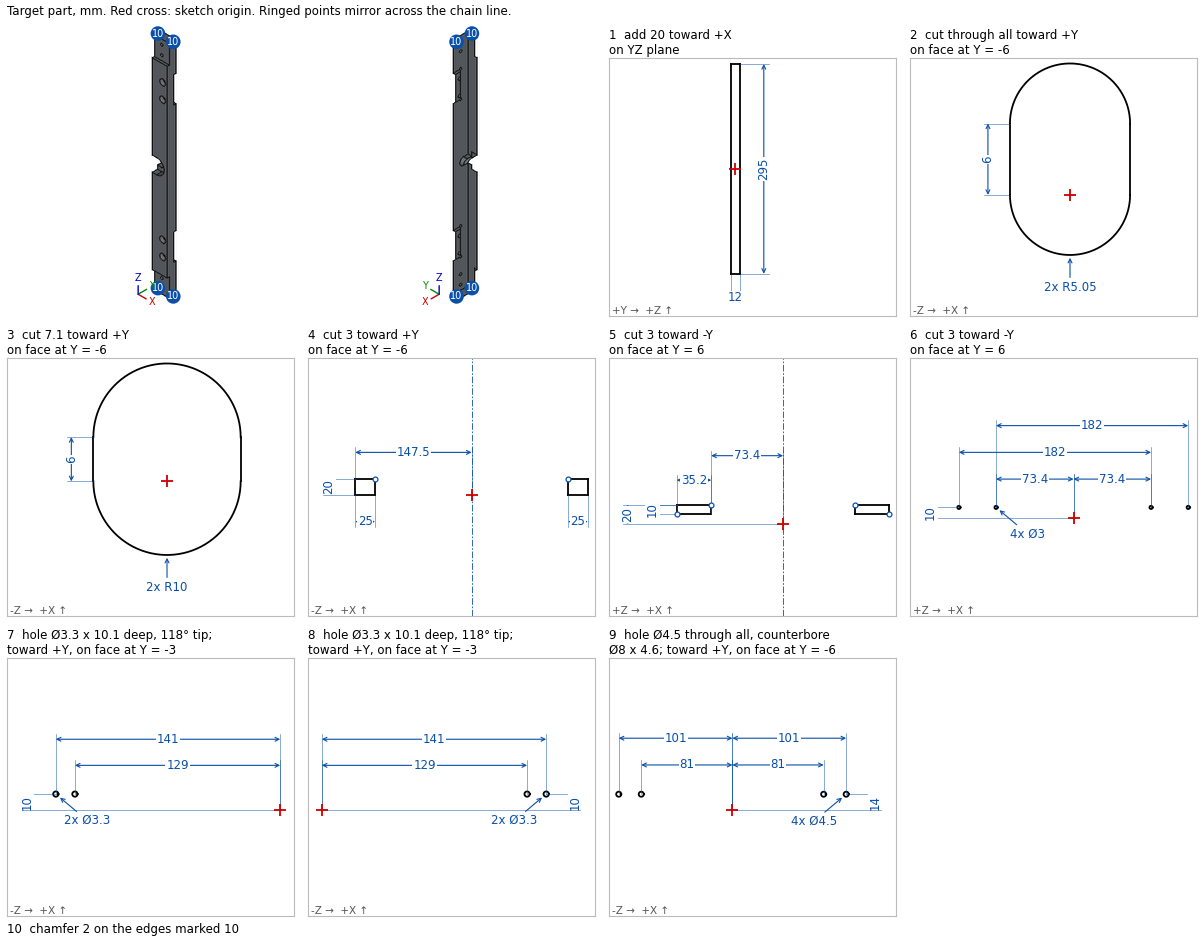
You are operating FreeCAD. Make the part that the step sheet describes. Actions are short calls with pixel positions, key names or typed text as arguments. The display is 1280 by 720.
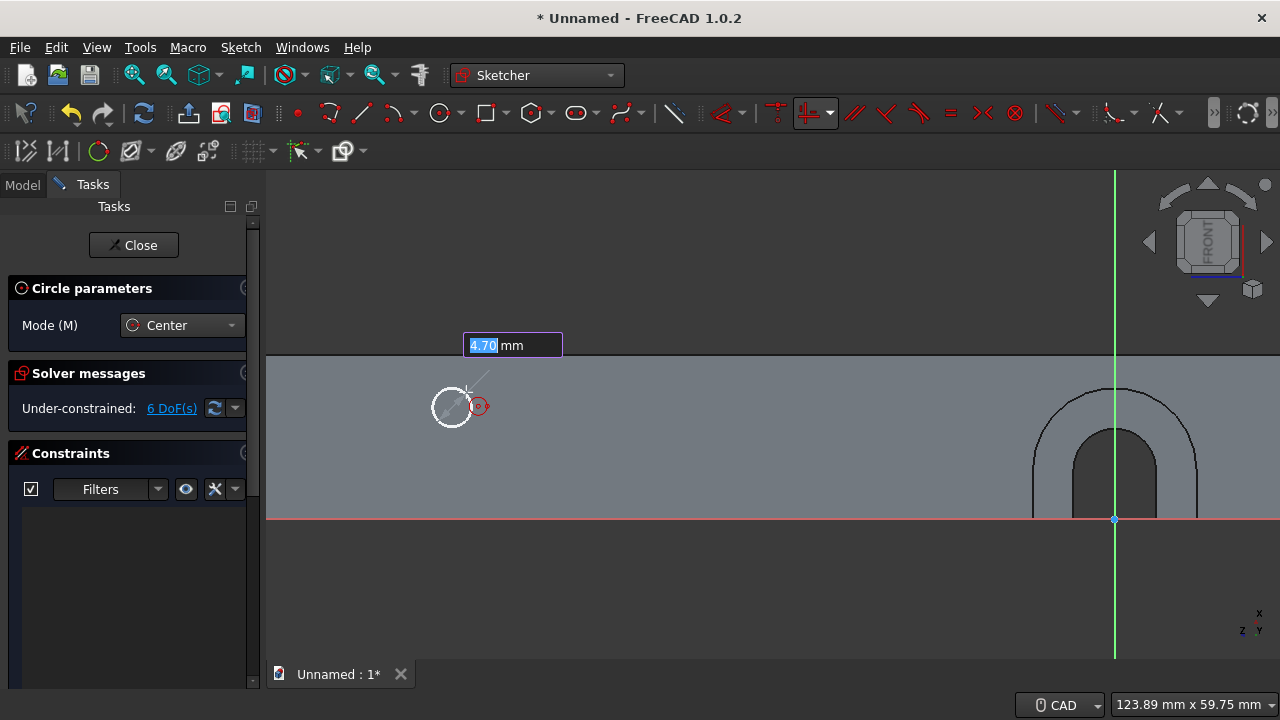
click(465, 391)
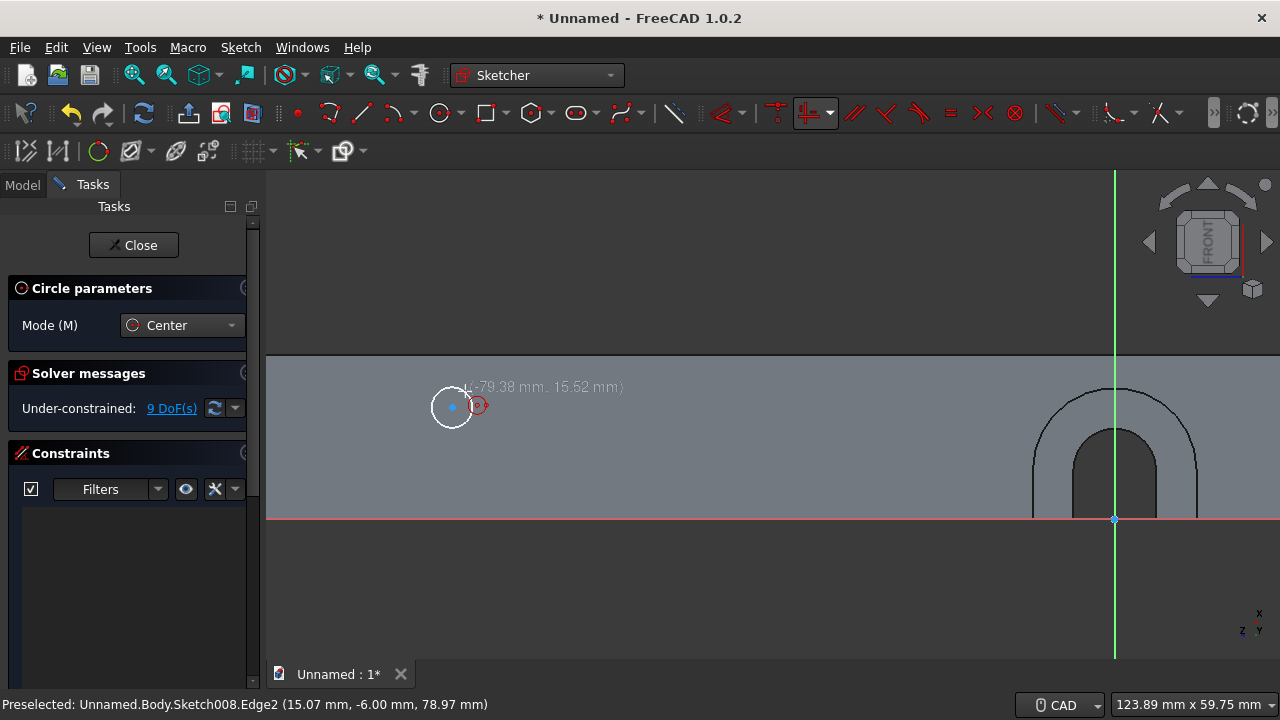
scroll(466, 392, down, 5)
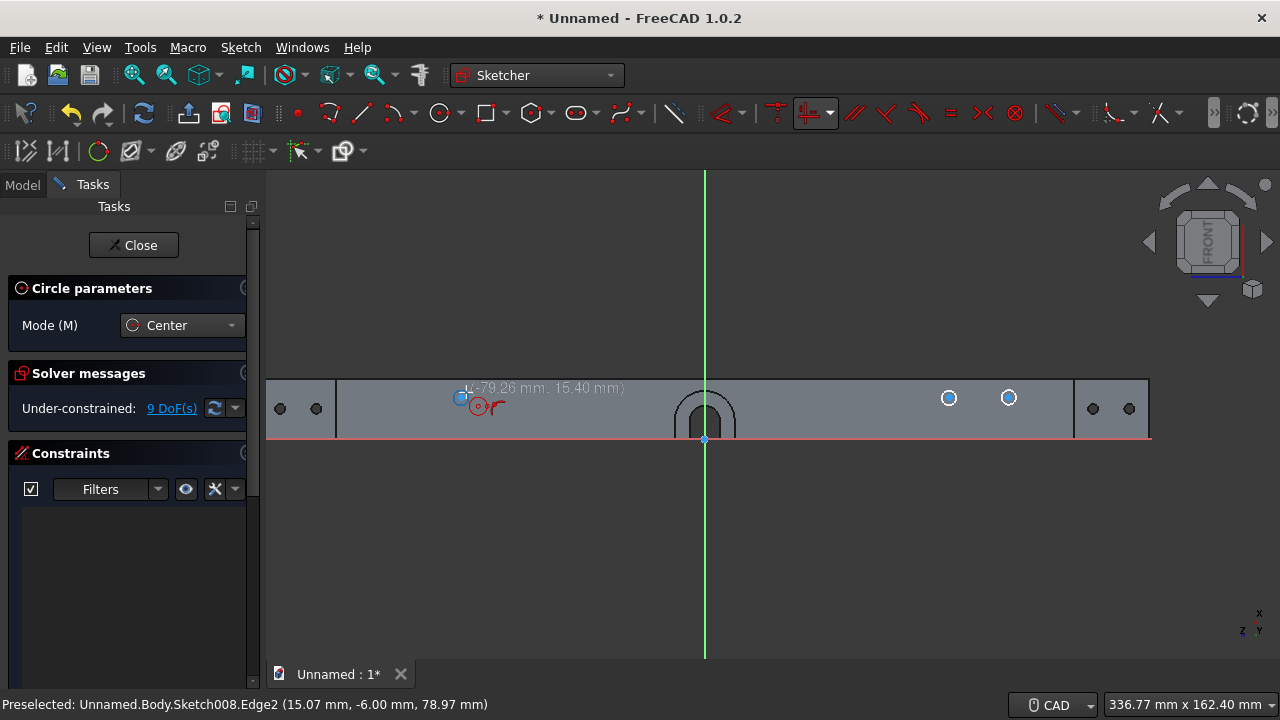
scroll(401, 397, up, 7)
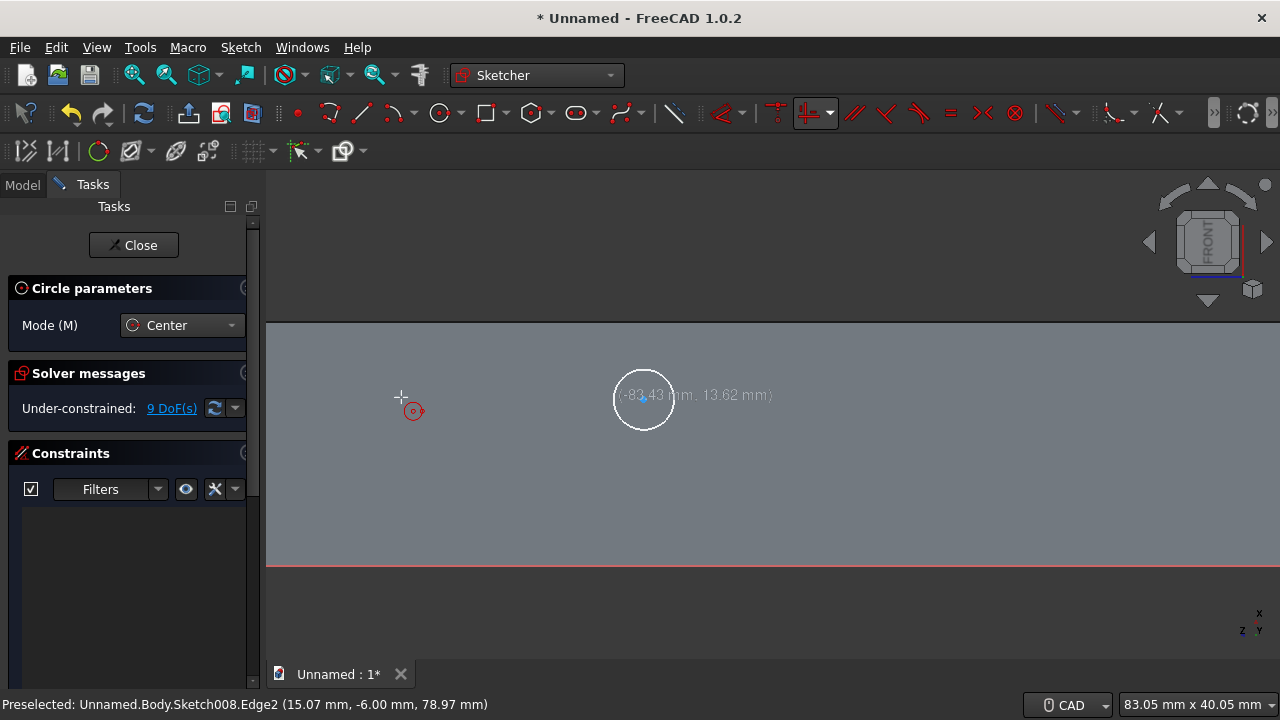
scroll(401, 397, down, 7)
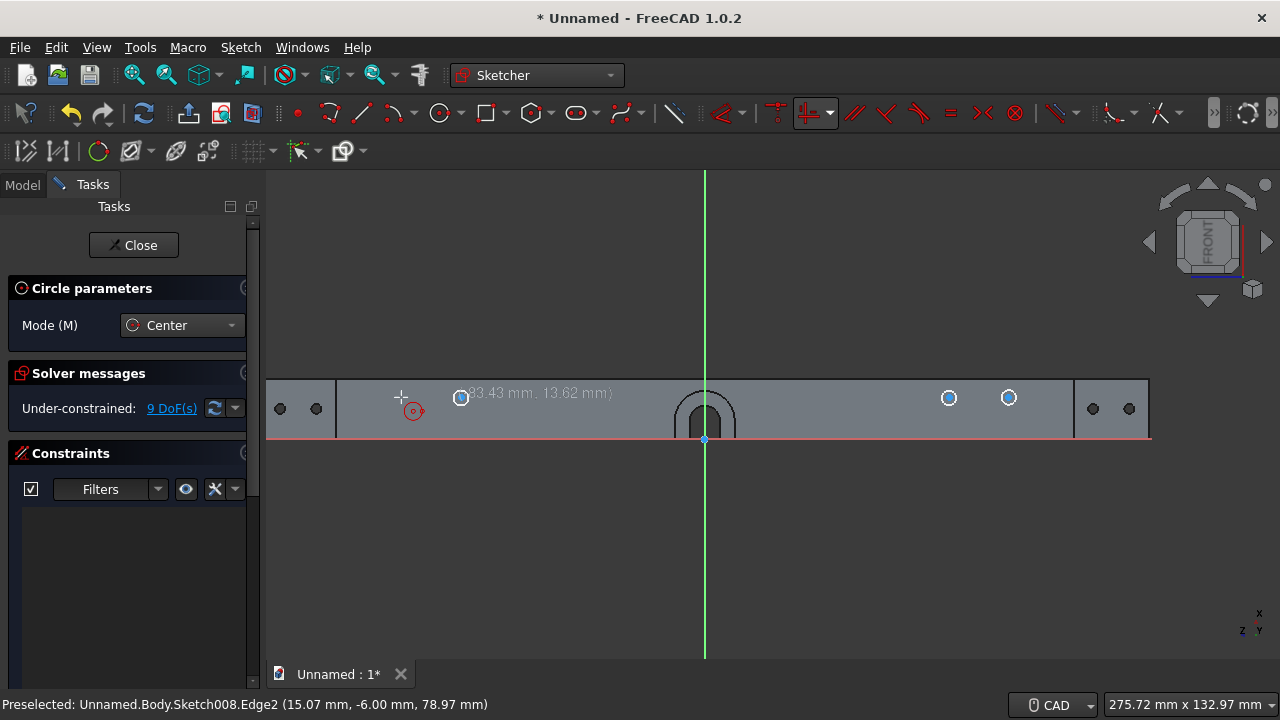
click(401, 397)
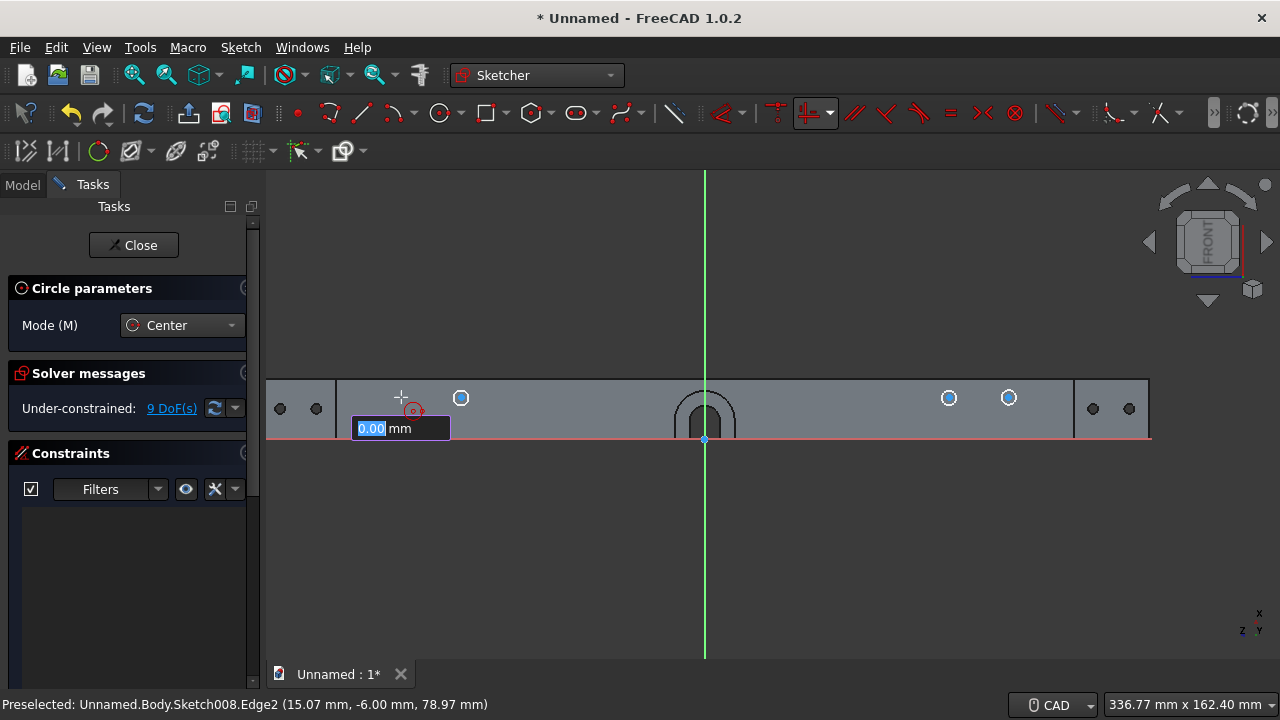
scroll(405, 392, up, 5)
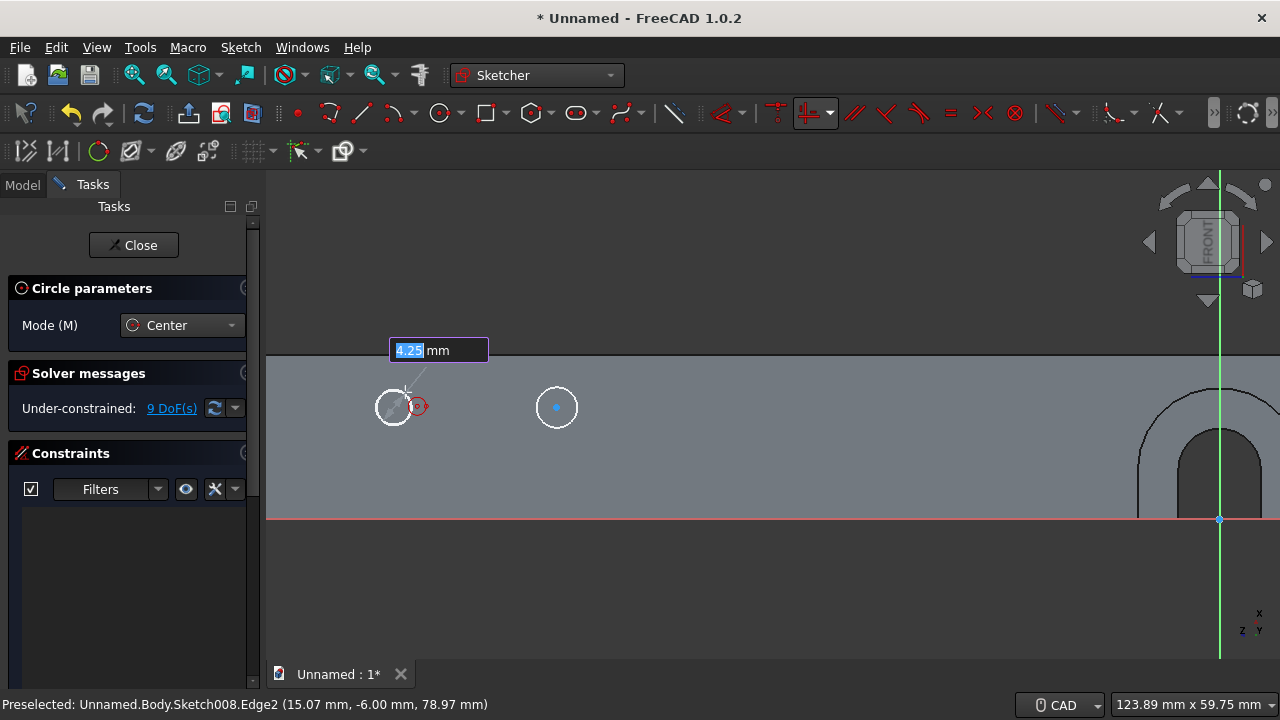
click(406, 391)
key(Escape)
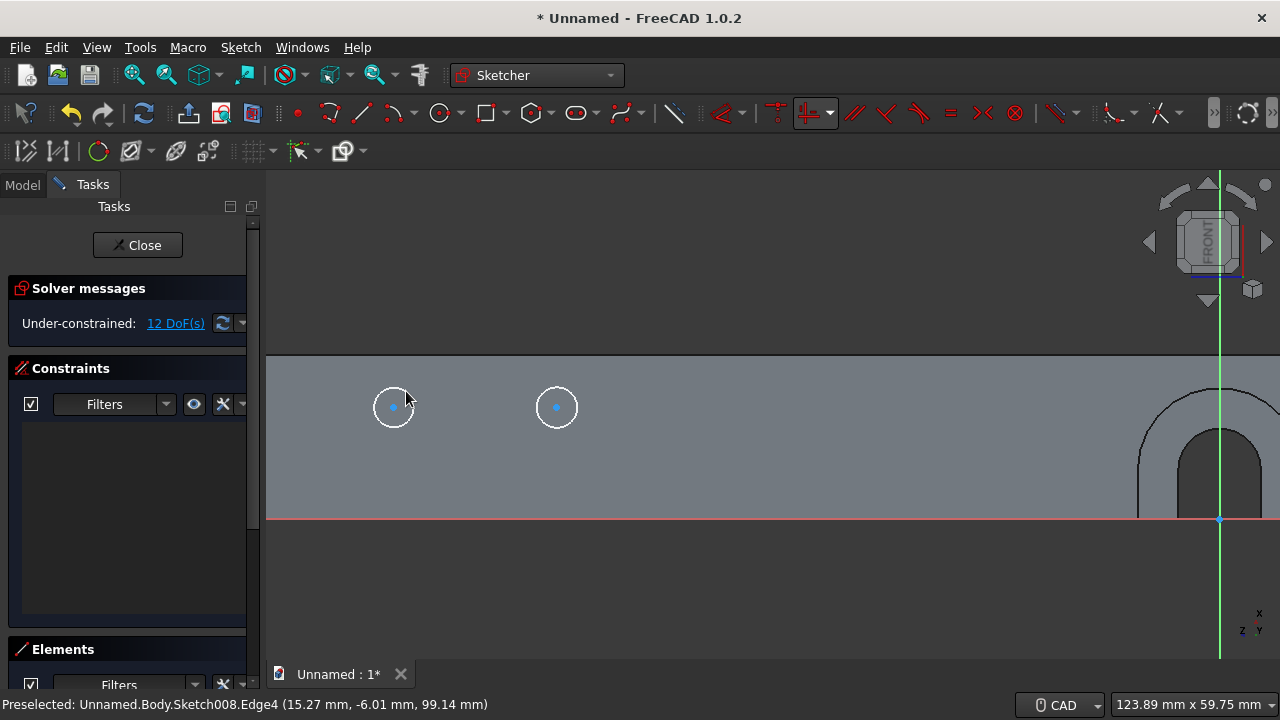
scroll(405, 392, down, 5)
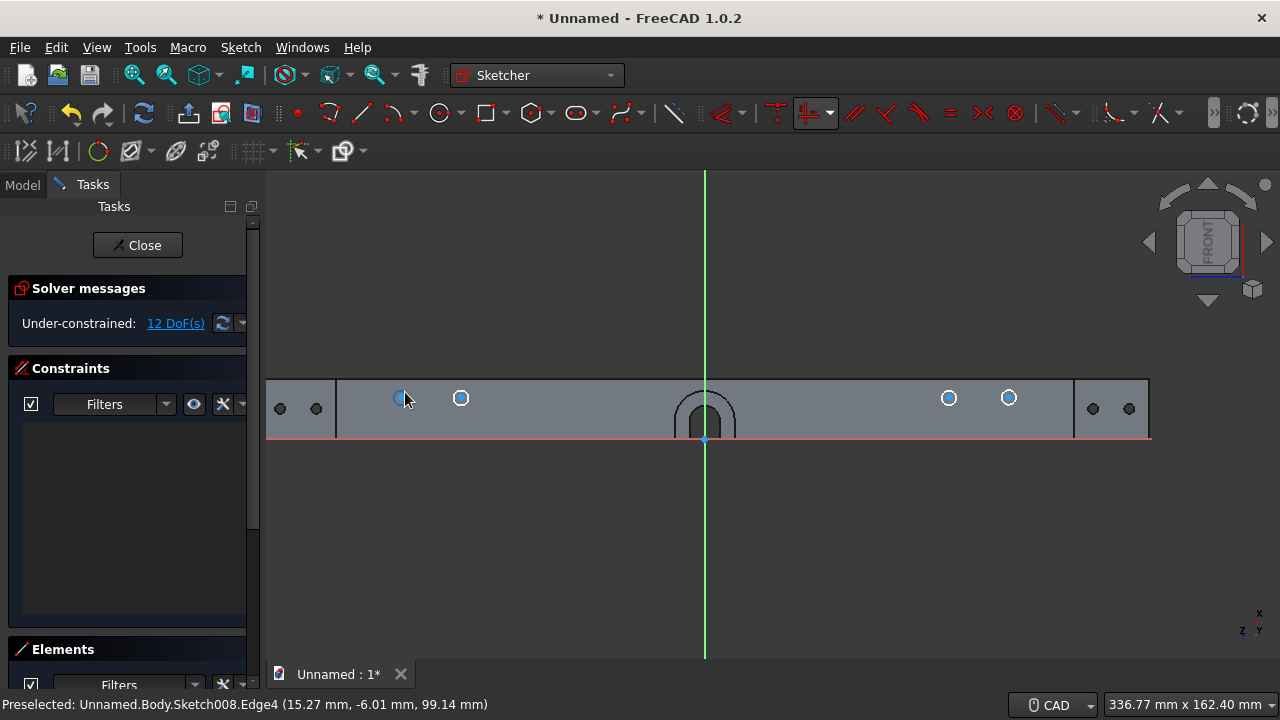
scroll(1014, 392, up, 4)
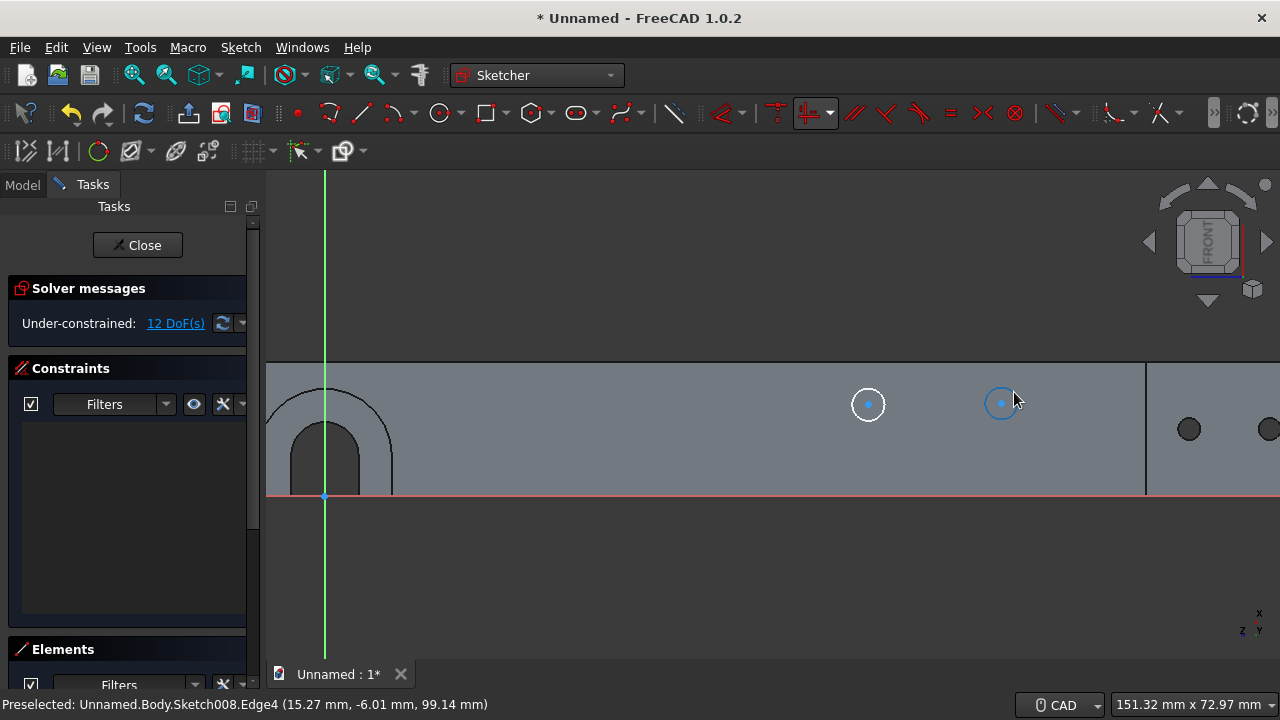
click(1013, 392)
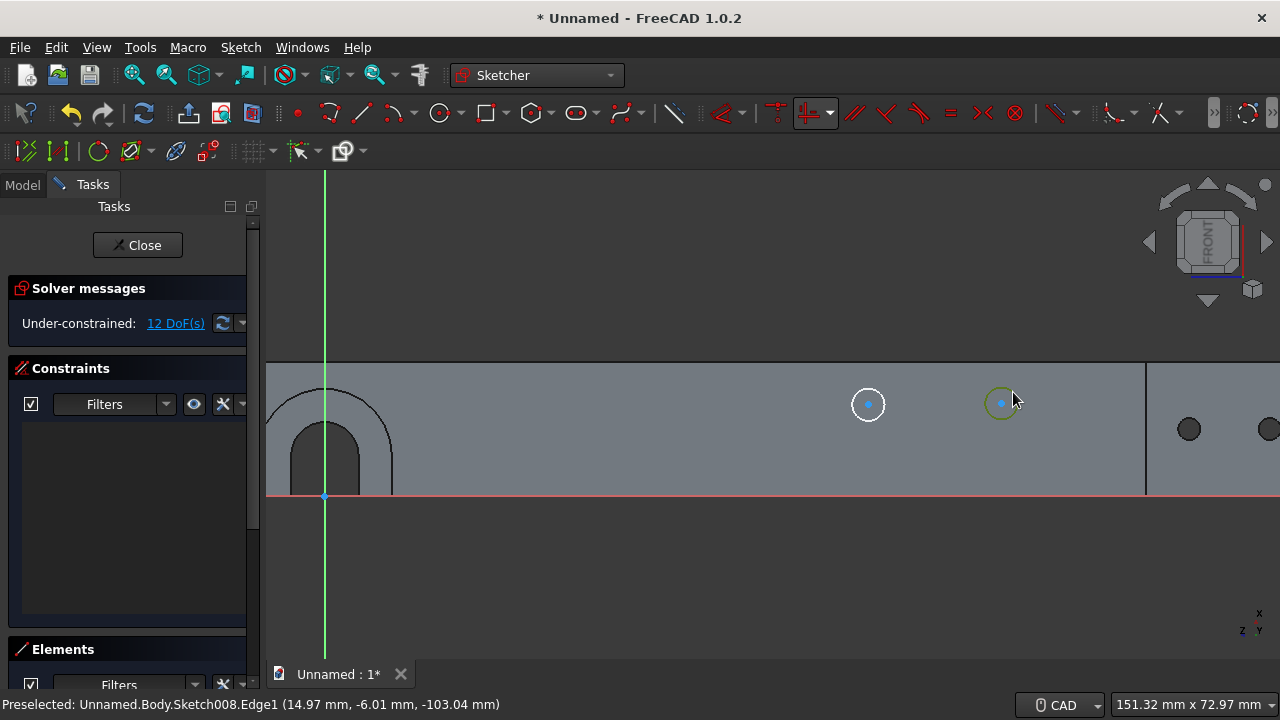
click(880, 393)